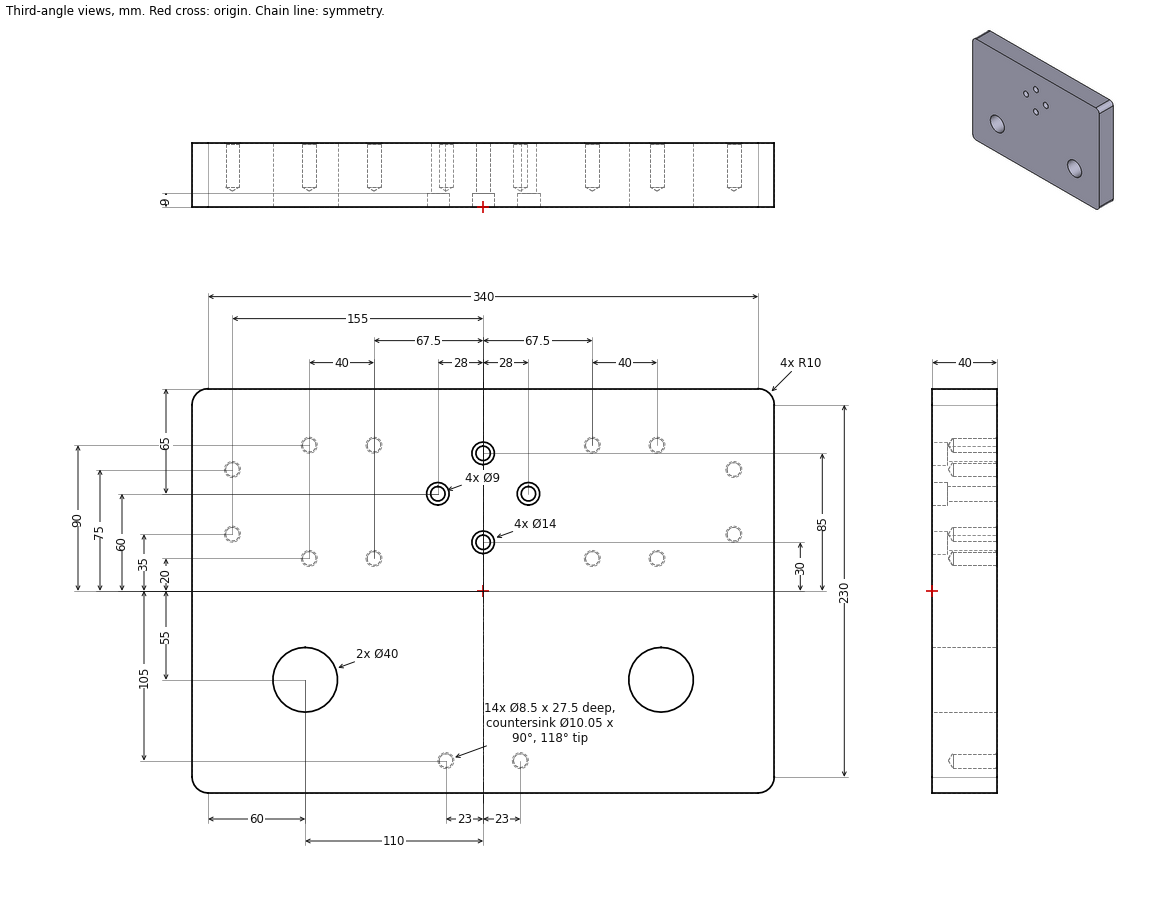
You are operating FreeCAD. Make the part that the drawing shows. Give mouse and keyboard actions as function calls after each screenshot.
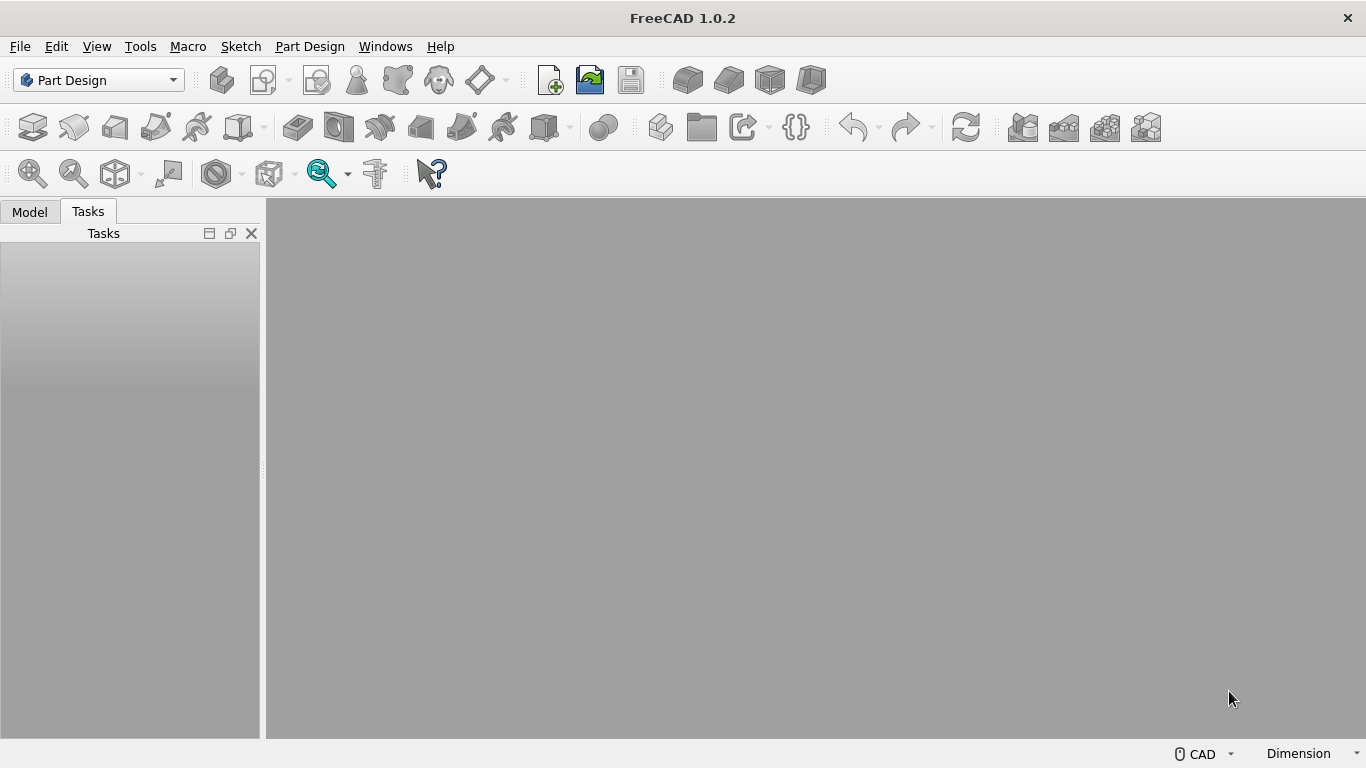
click(549, 80)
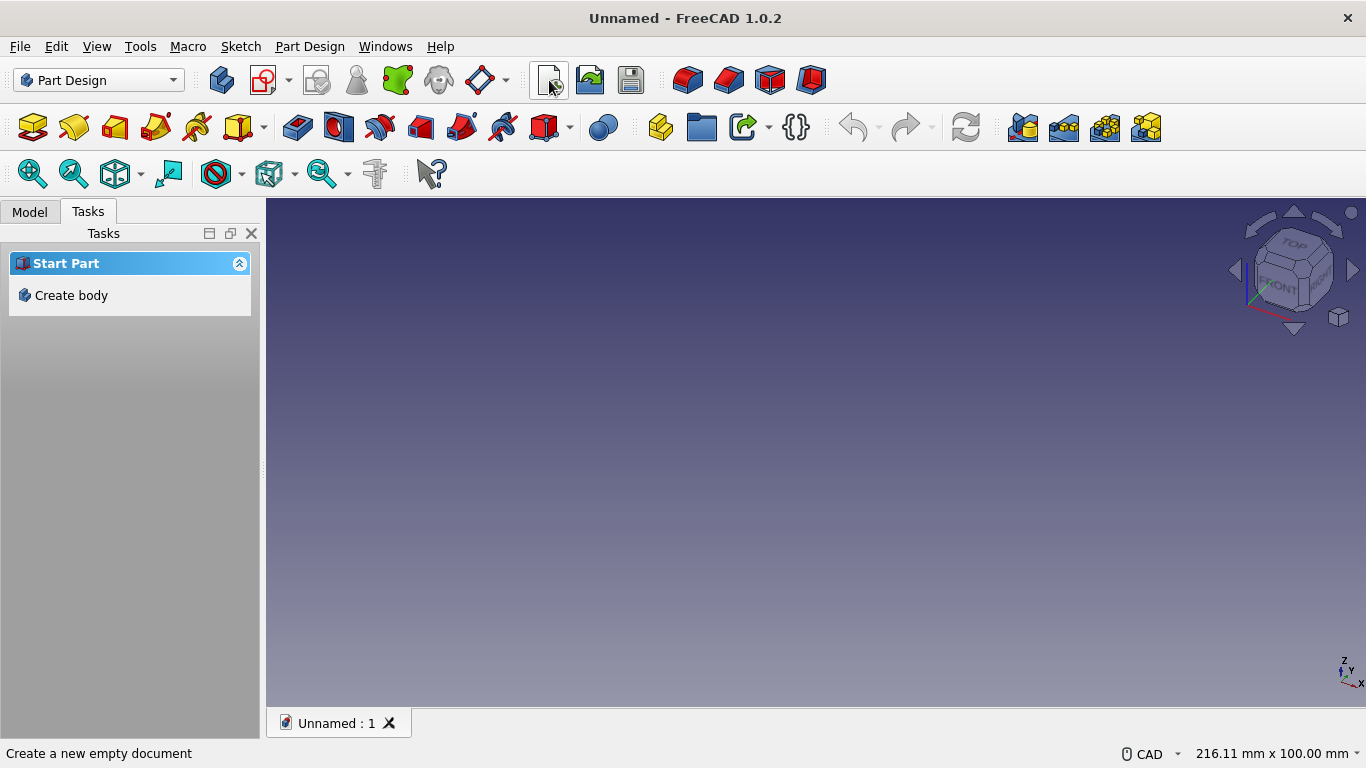
click(262, 80)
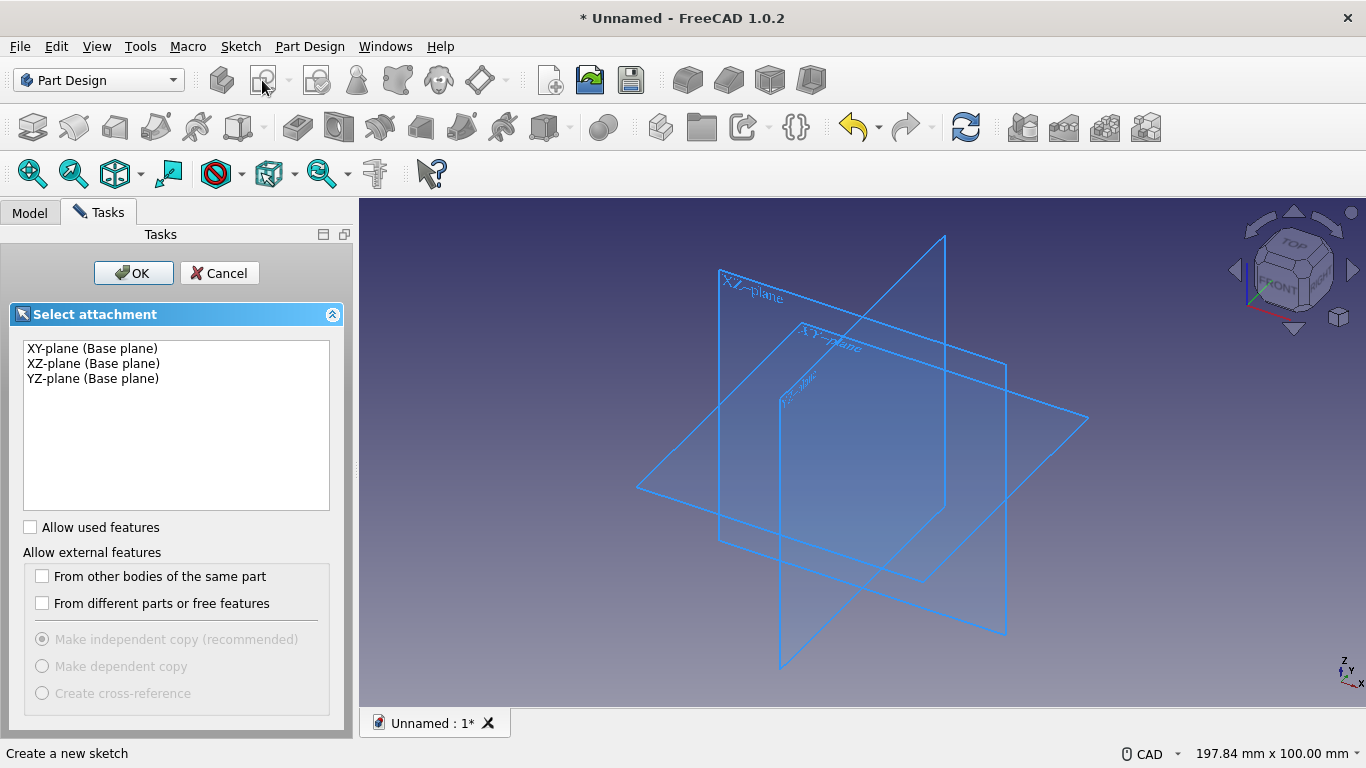
click(84, 364)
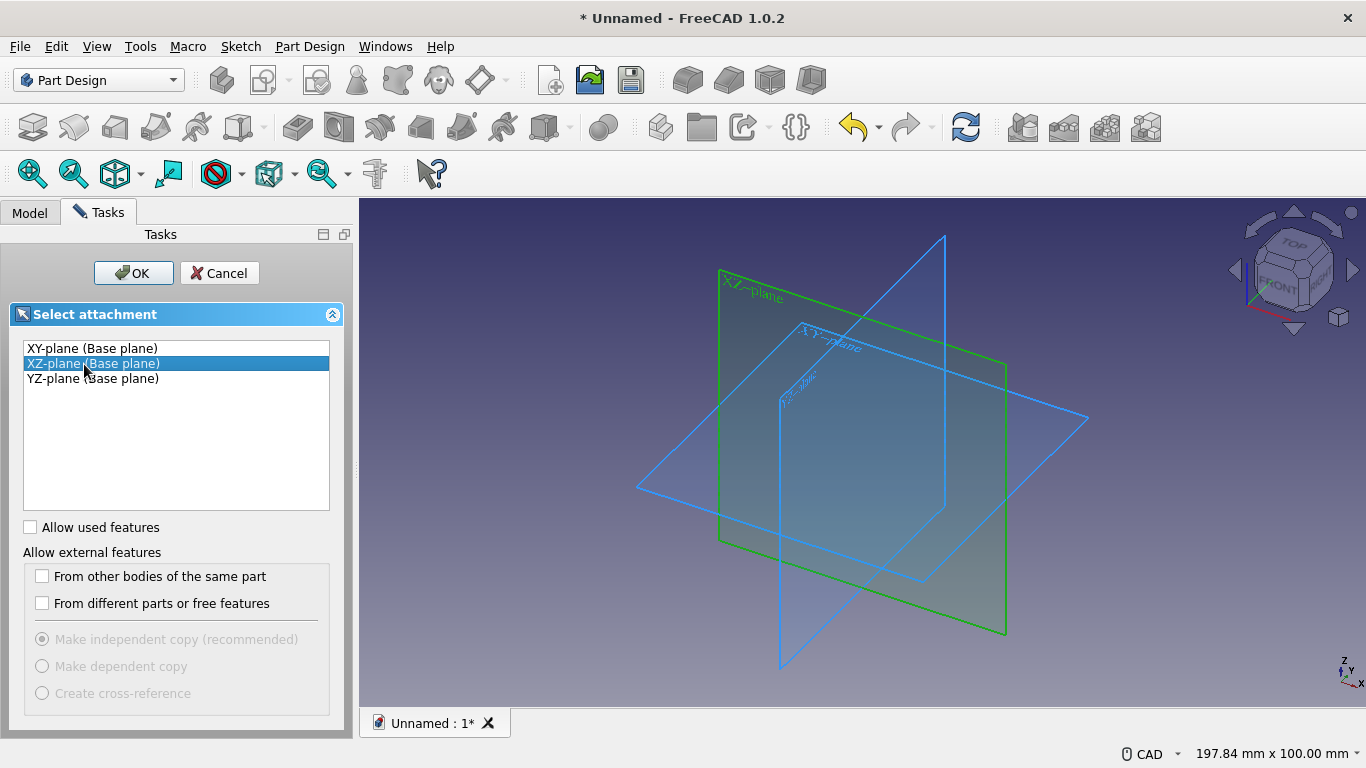
click(134, 273)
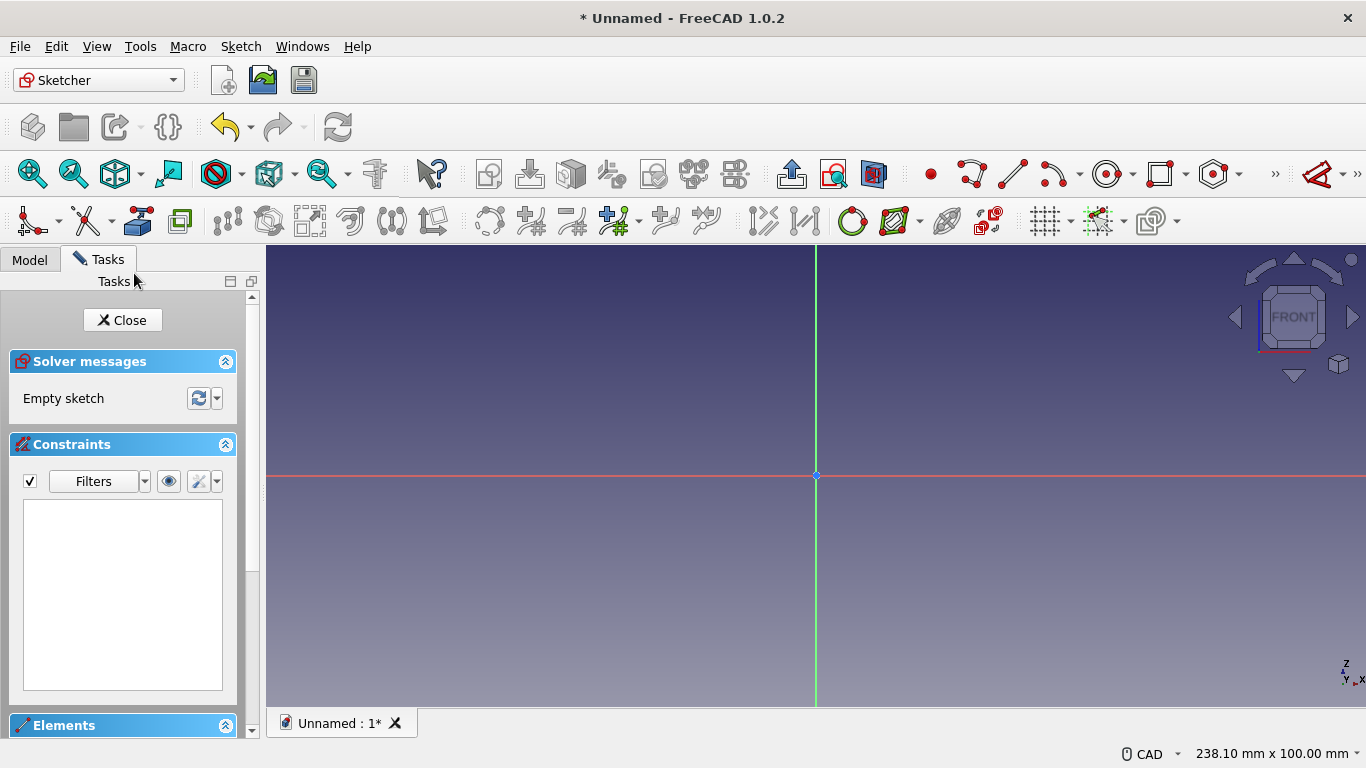
scroll(725, 476, down, 7)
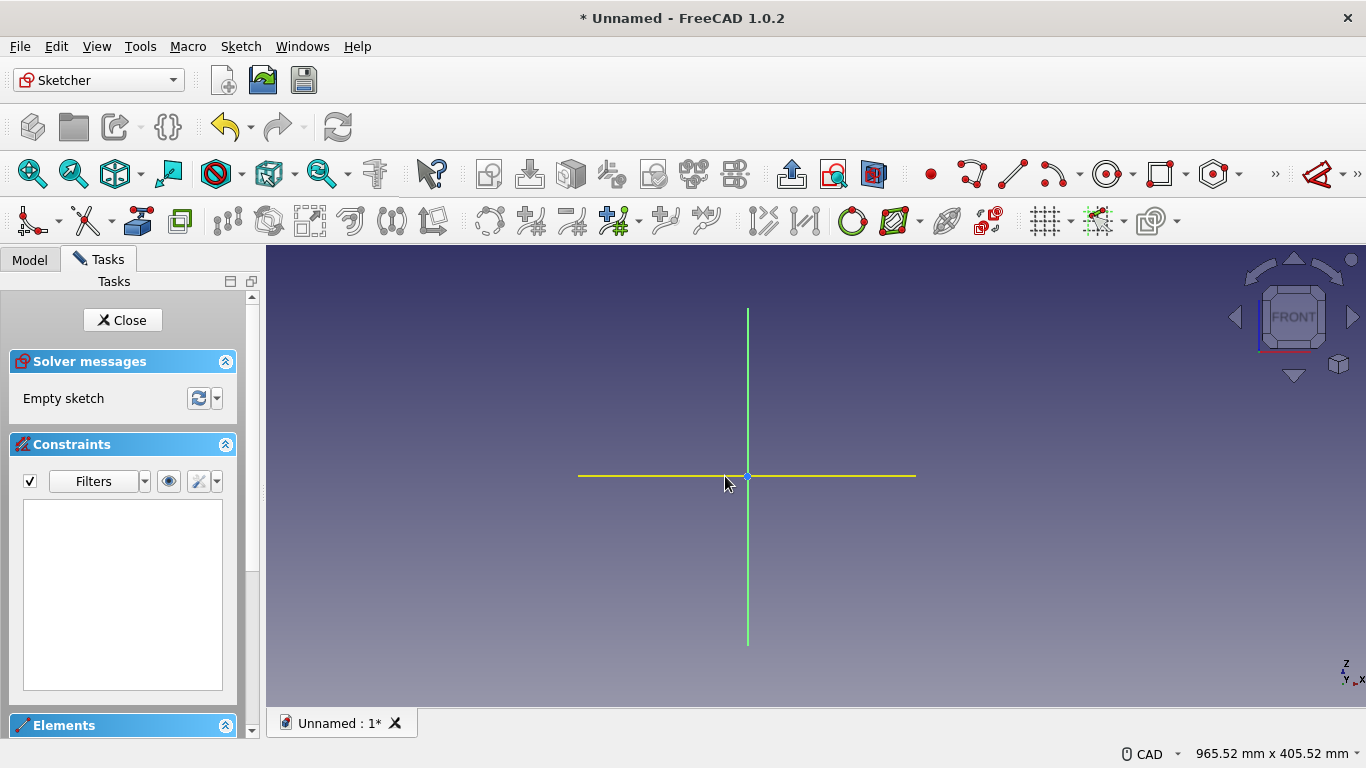
click(1013, 174)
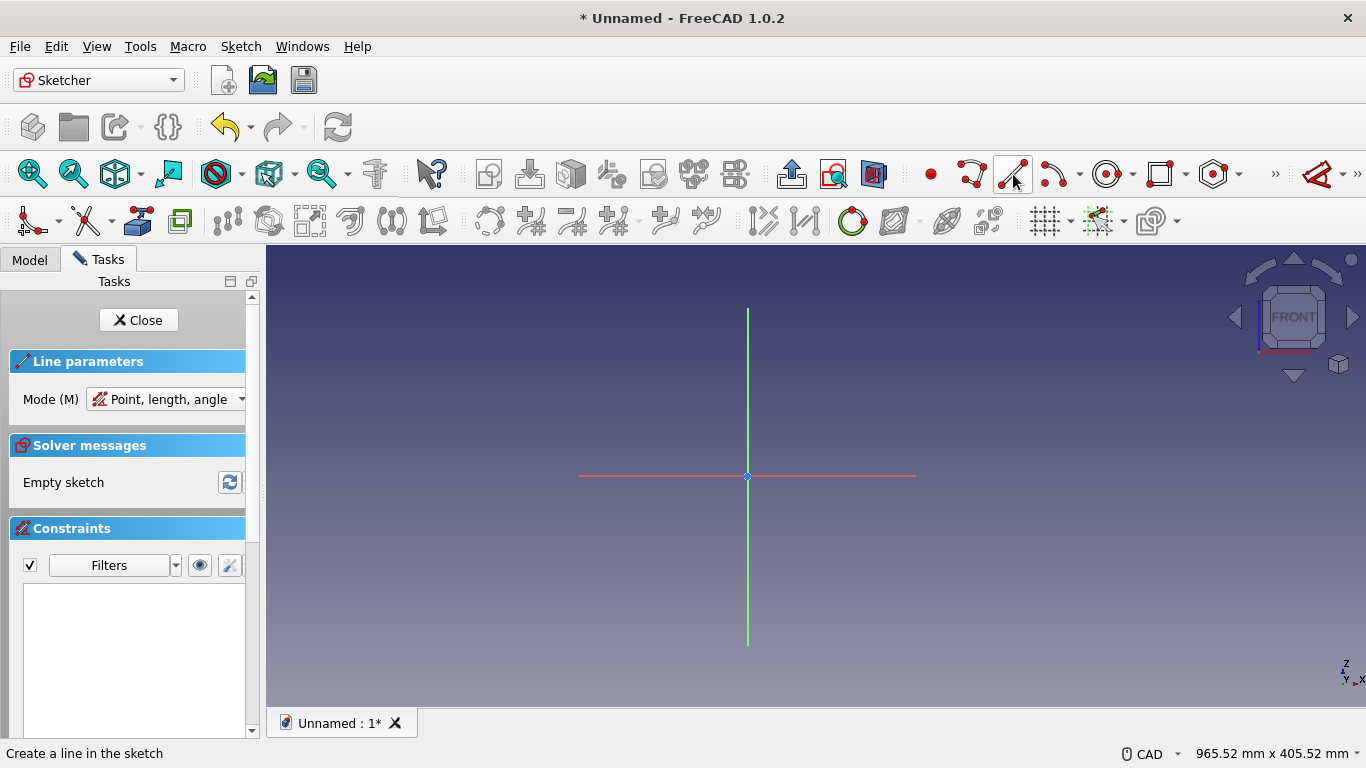
click(554, 334)
click(941, 334)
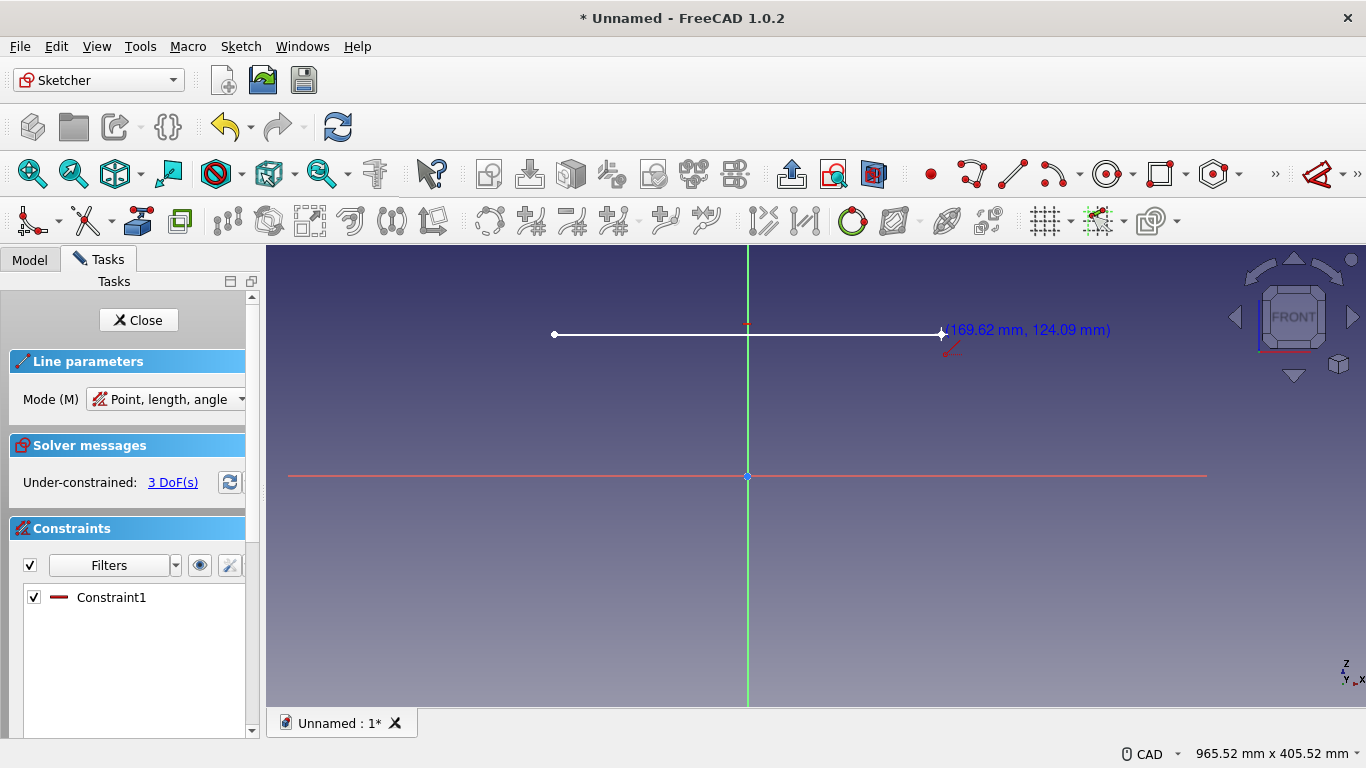
click(953, 345)
click(953, 607)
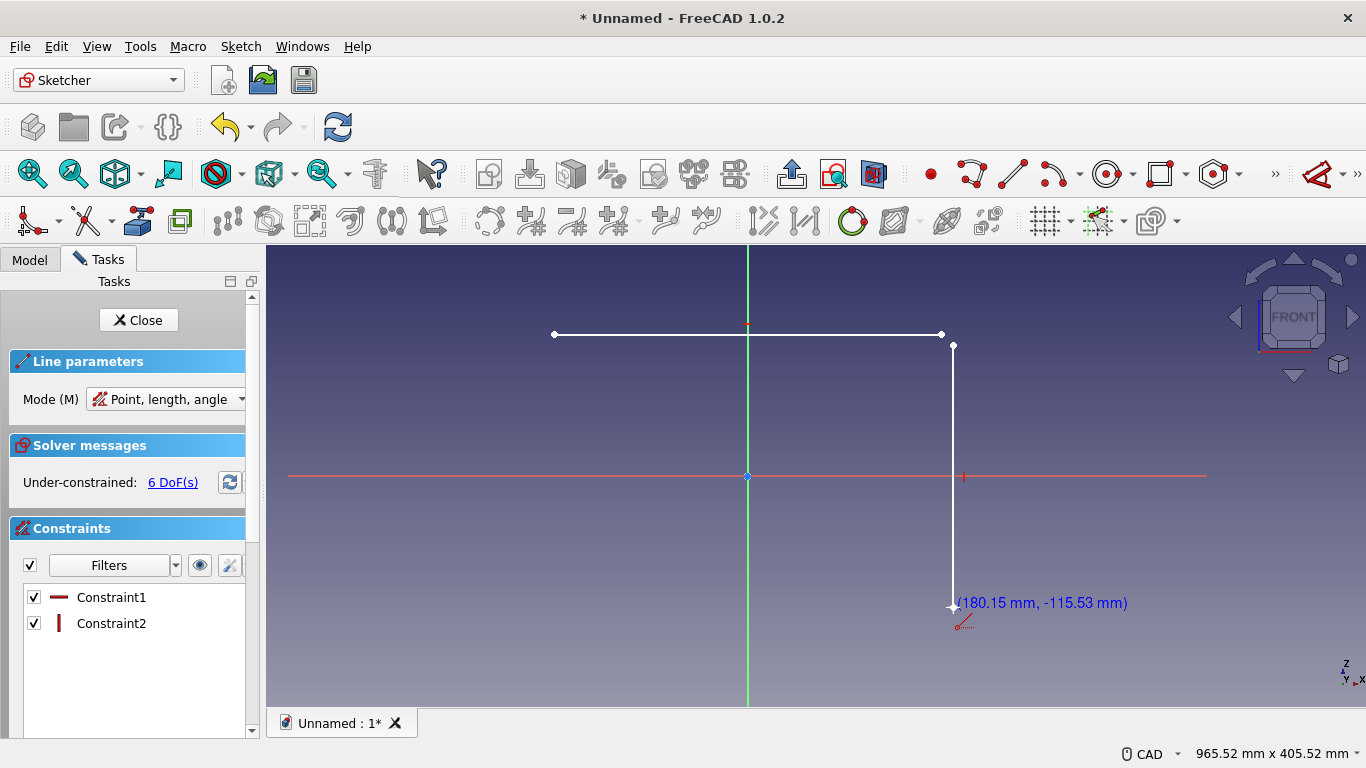
click(941, 619)
click(554, 619)